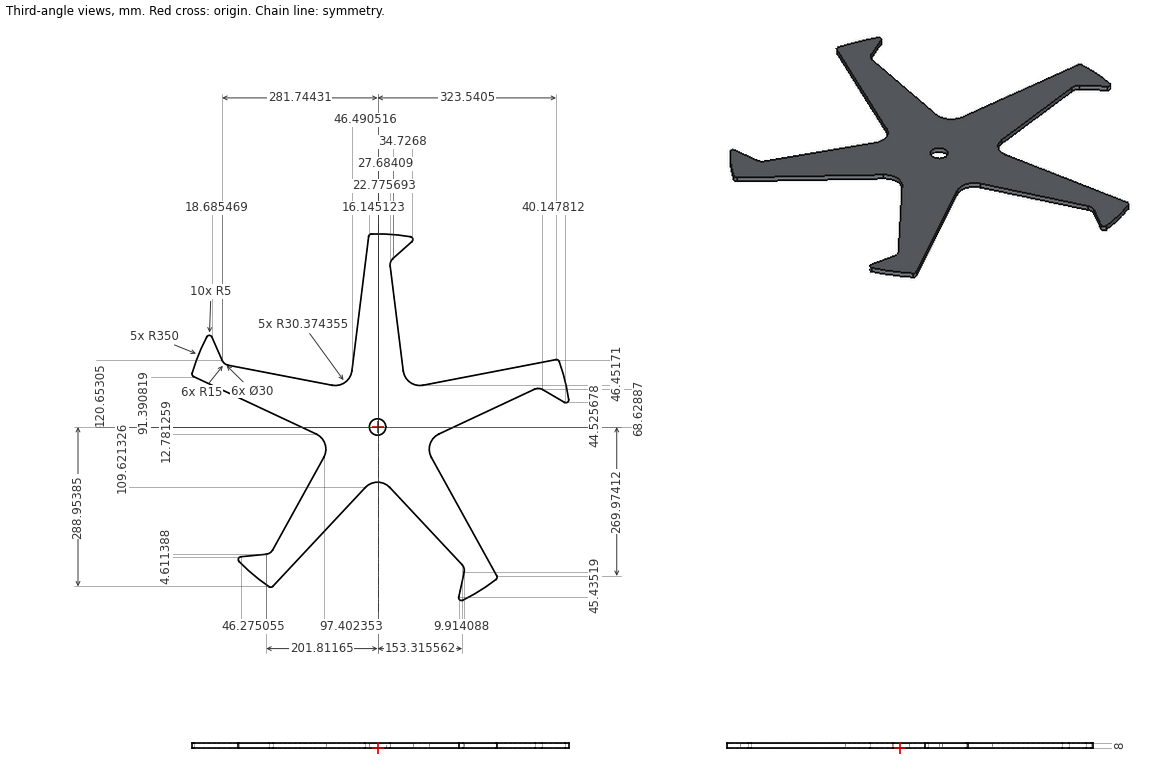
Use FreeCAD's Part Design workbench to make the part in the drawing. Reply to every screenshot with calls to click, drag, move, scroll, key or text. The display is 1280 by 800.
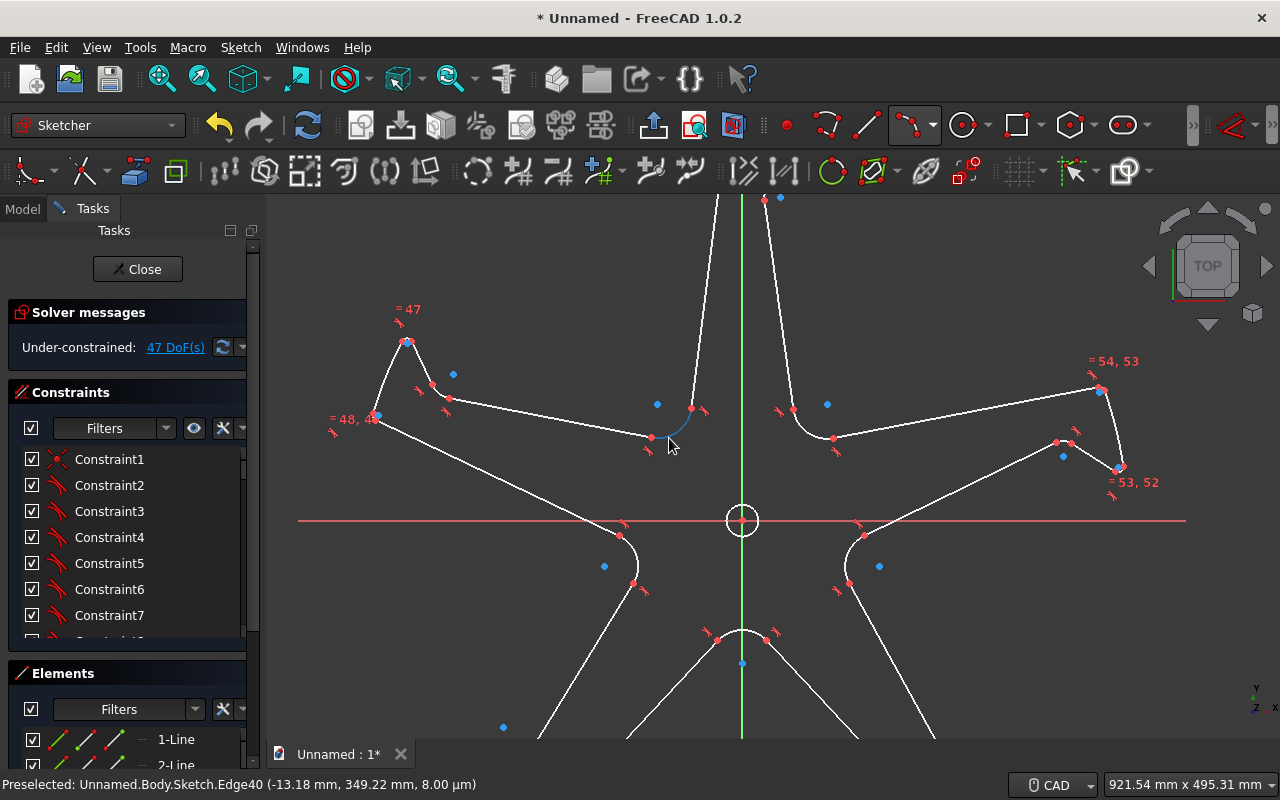
click(668, 437)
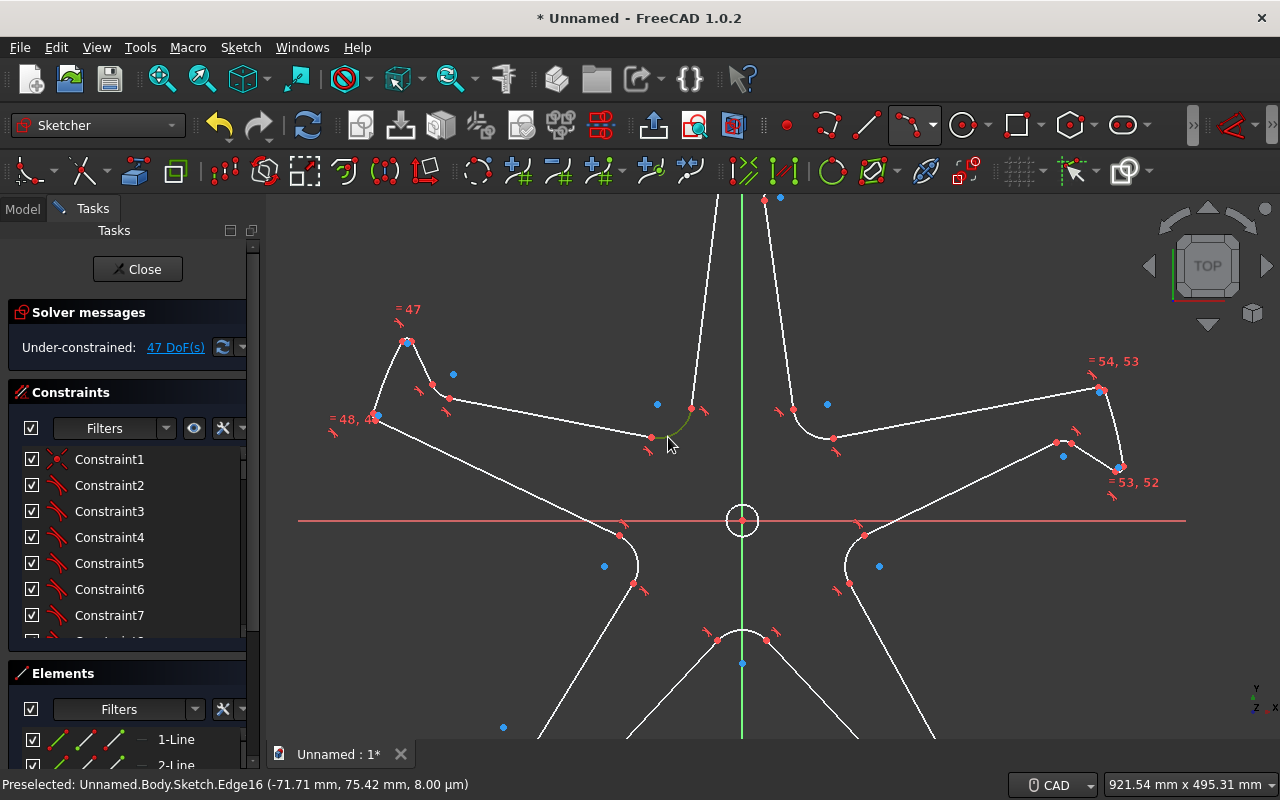
click(638, 568)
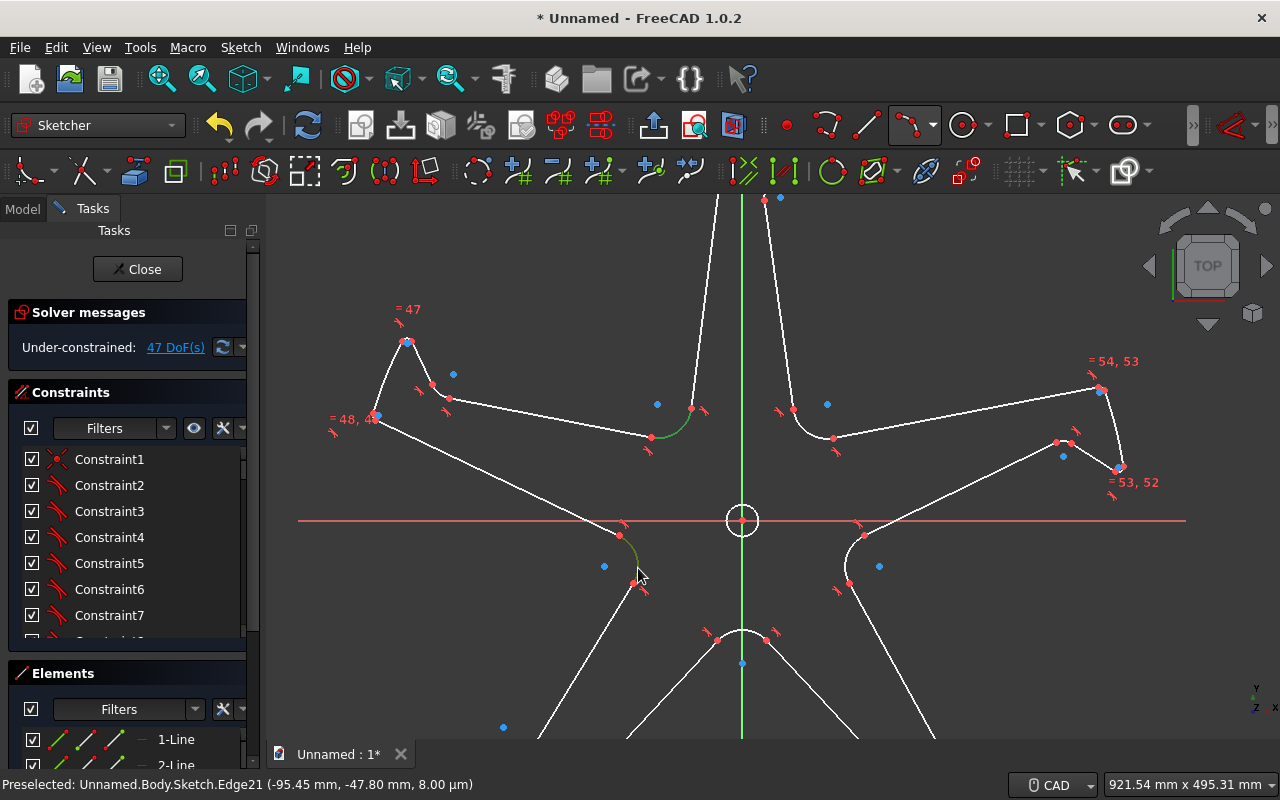
scroll(753, 632, up, 2)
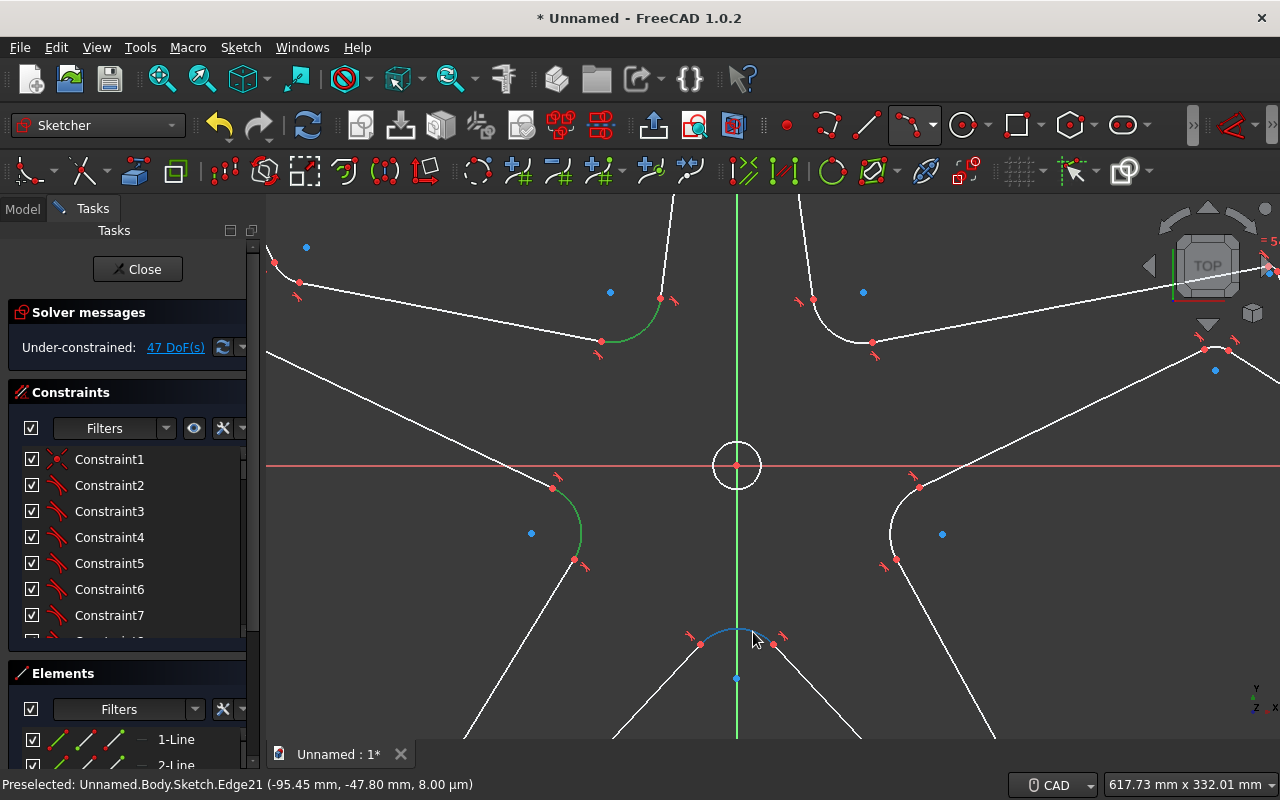
click(753, 631)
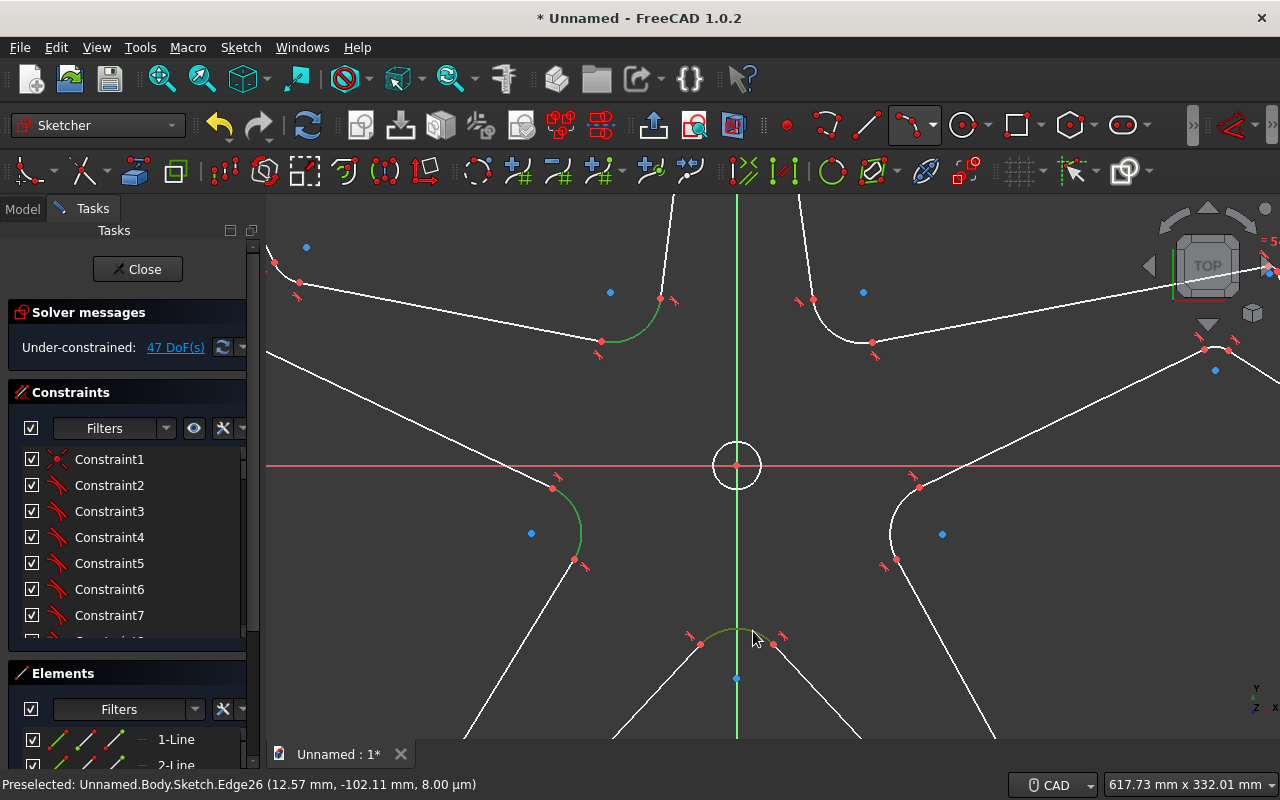
click(900, 504)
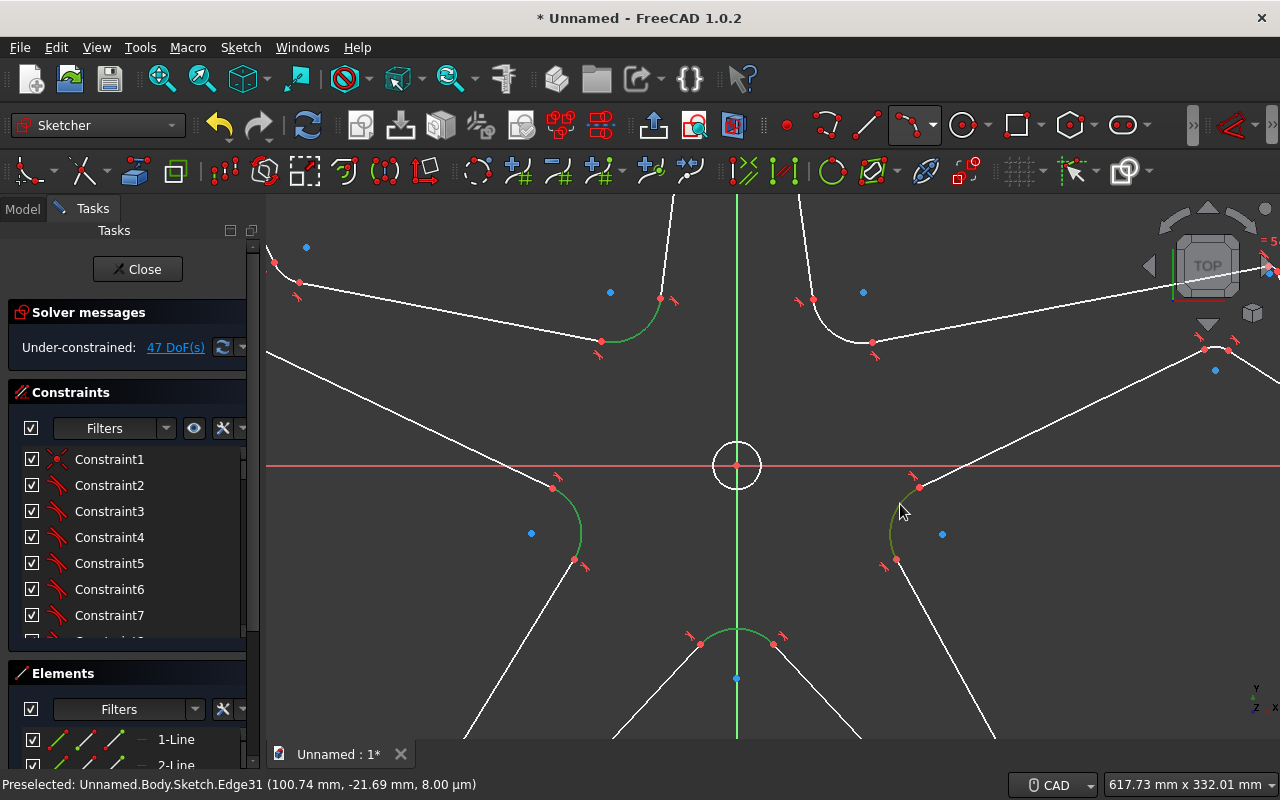
click(822, 322)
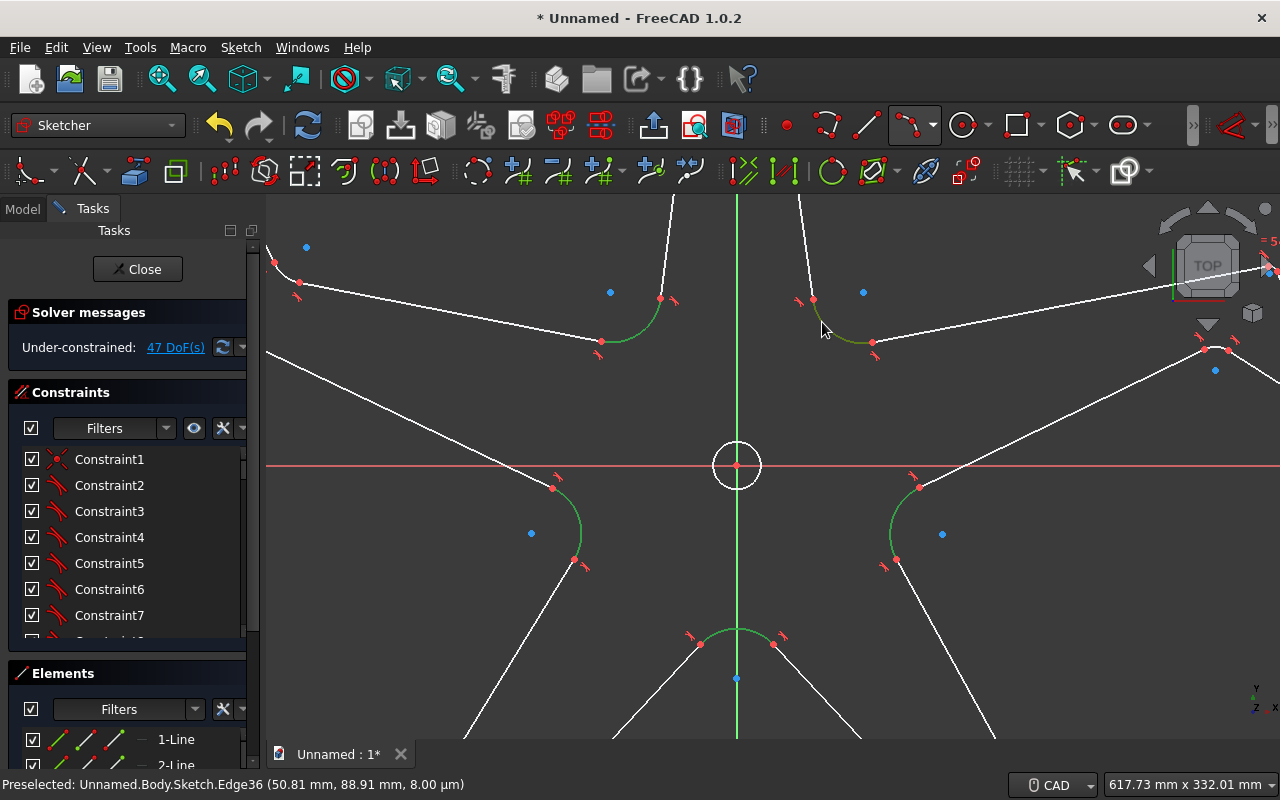
key(e)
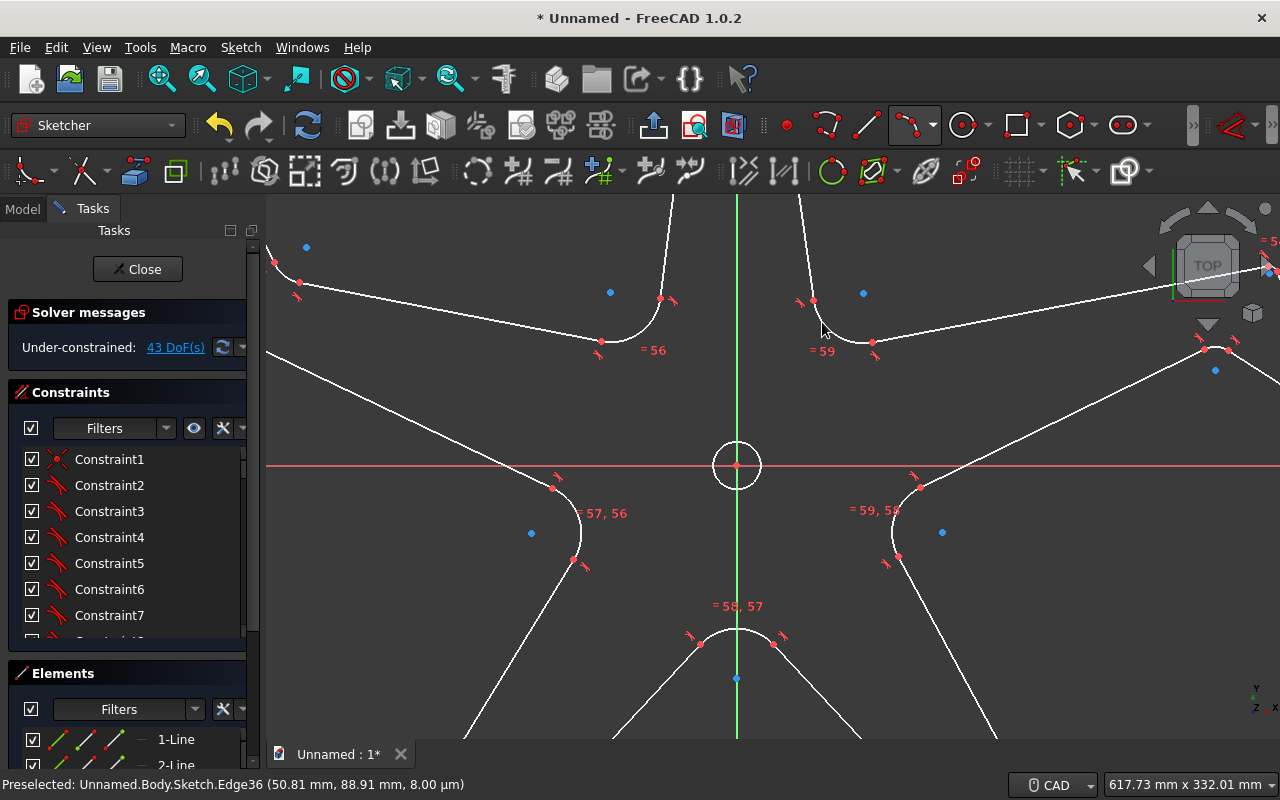
scroll(687, 479, down, 6)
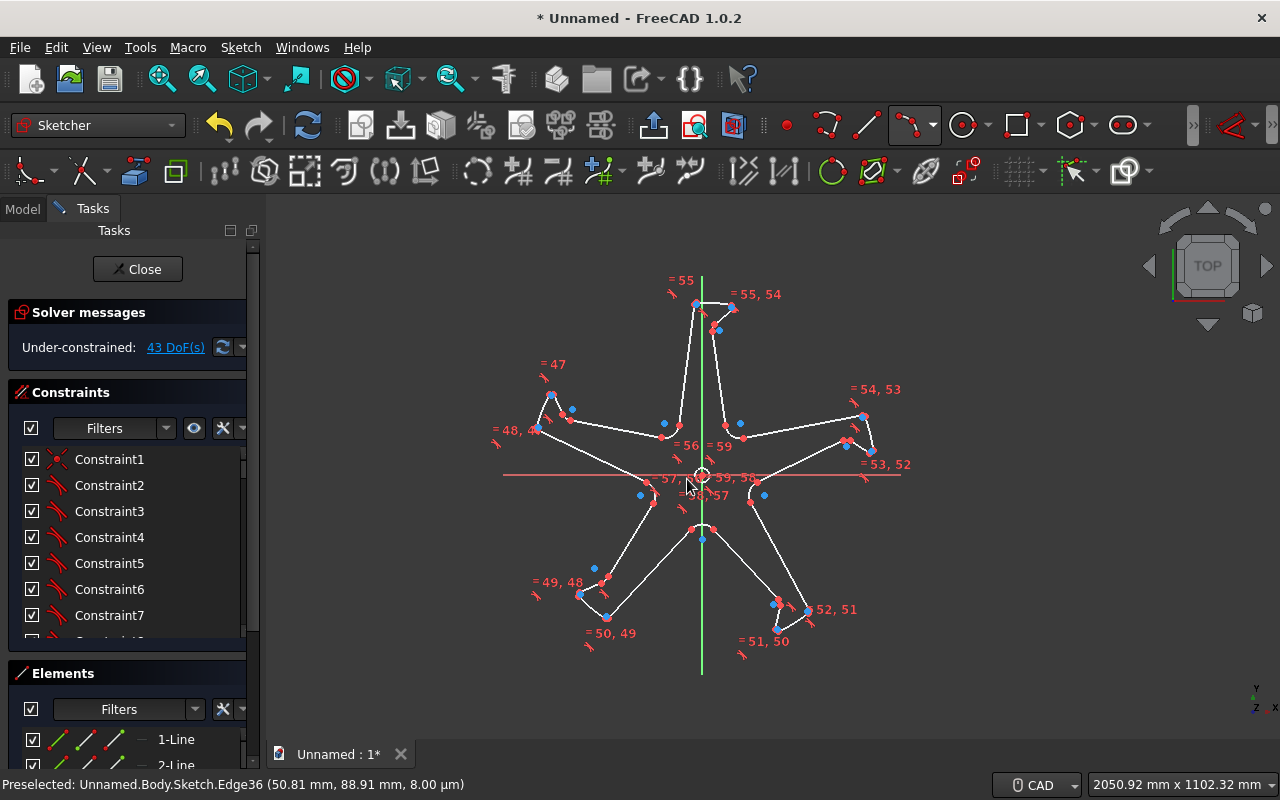
scroll(565, 417, up, 8)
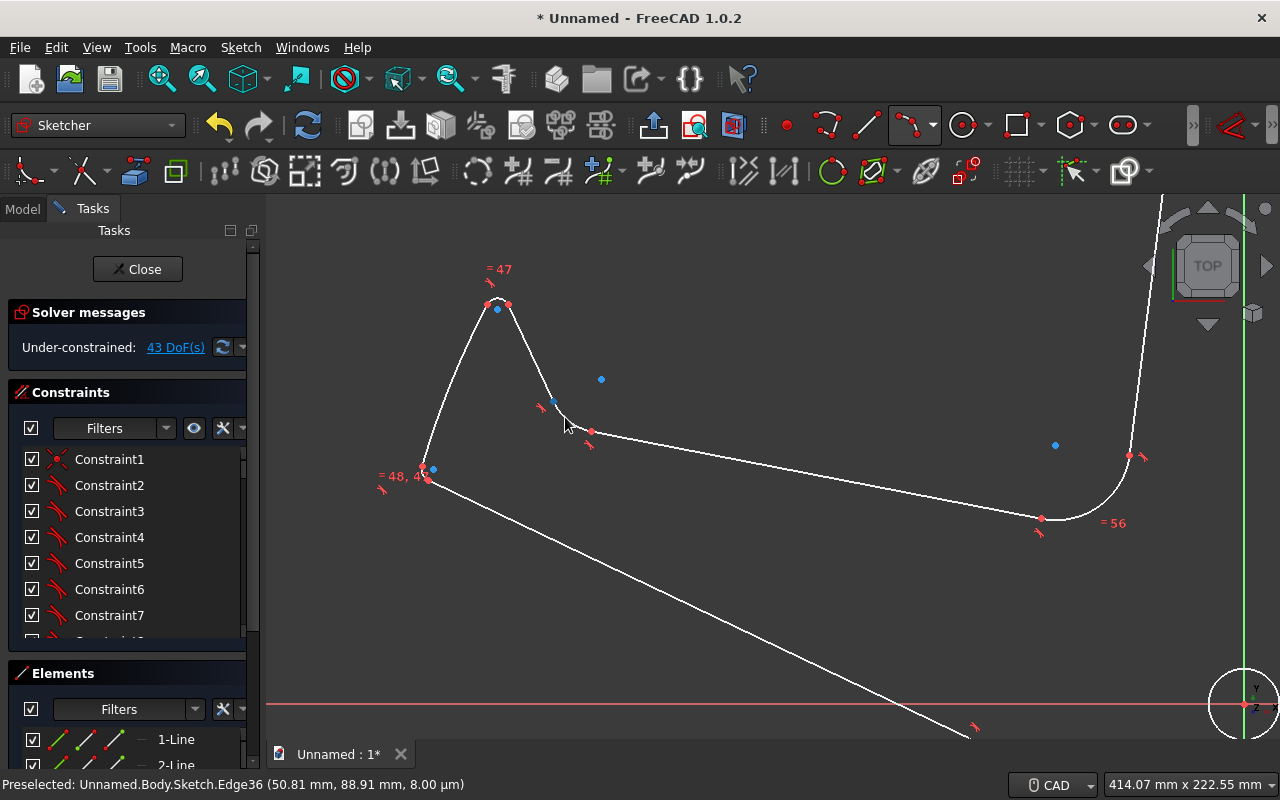
click(562, 414)